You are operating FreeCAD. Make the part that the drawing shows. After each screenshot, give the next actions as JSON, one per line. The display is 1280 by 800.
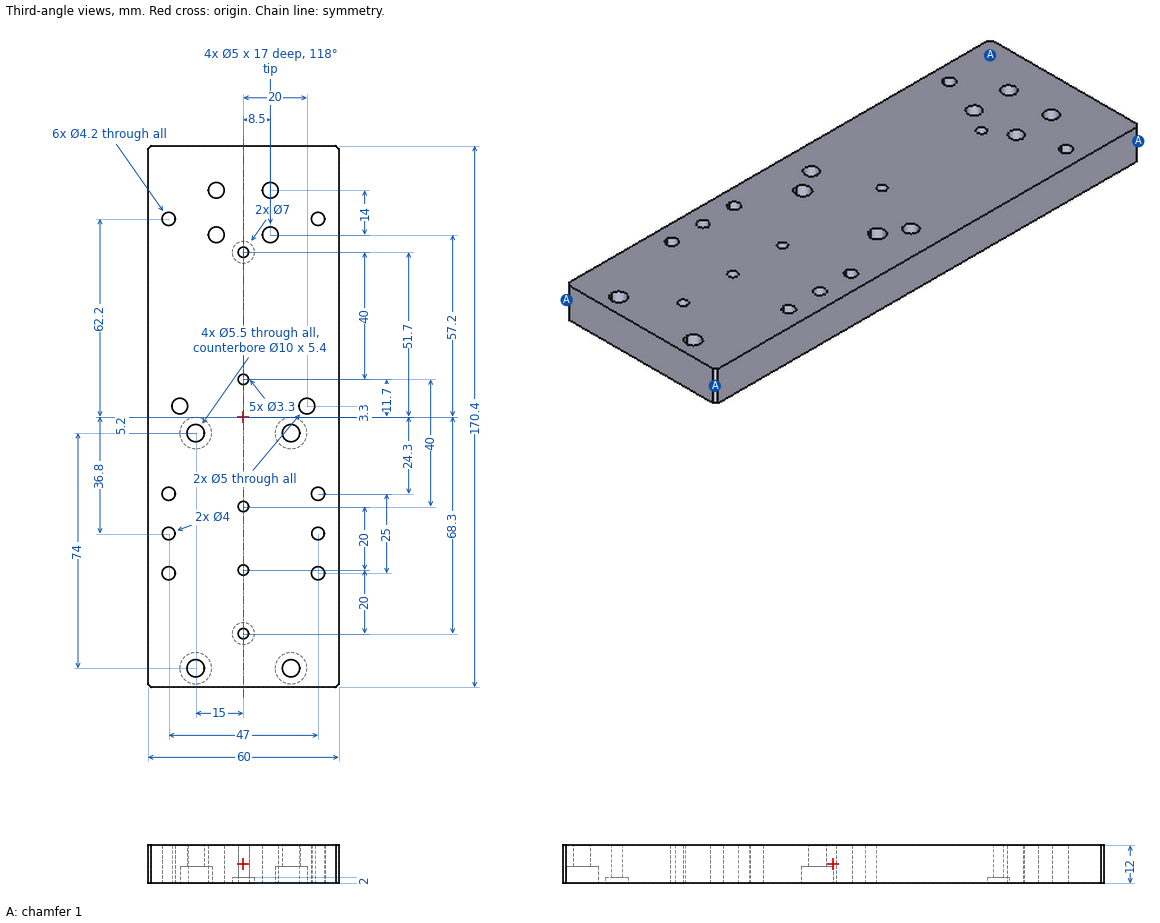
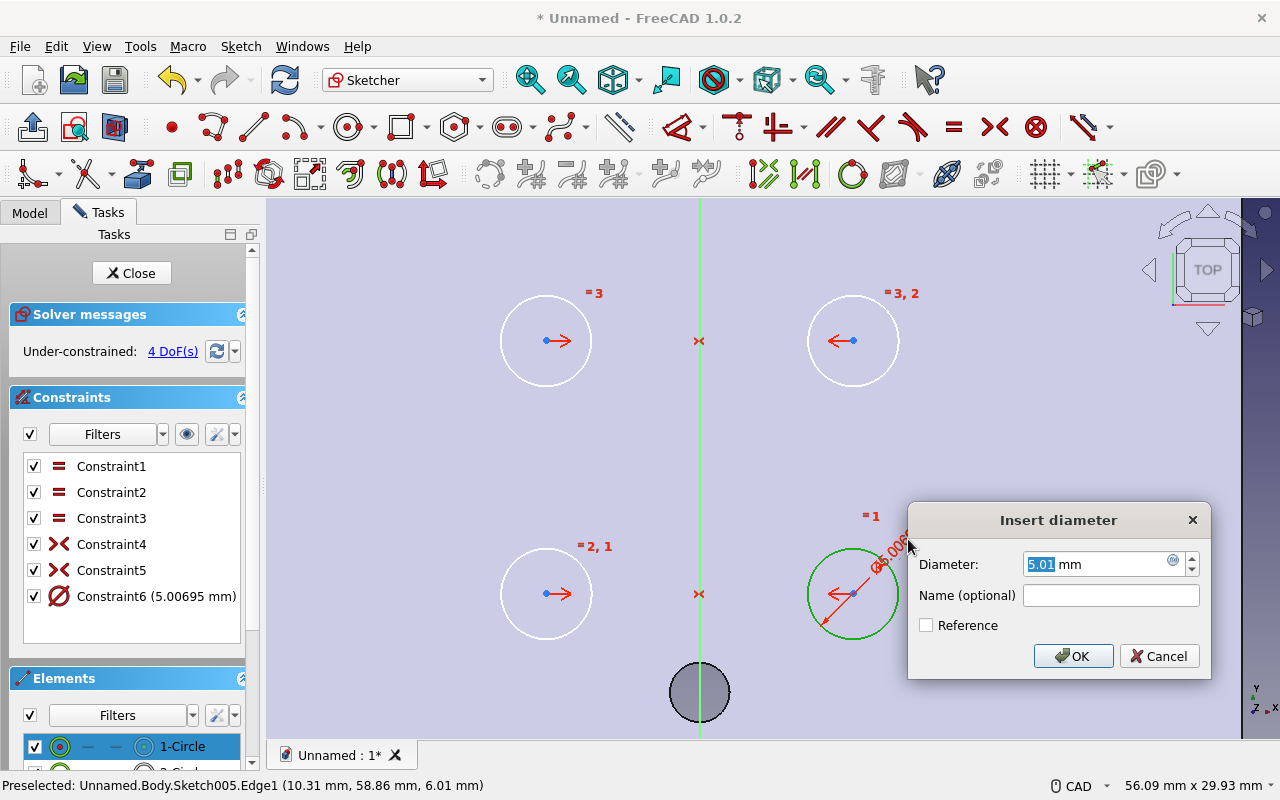
{"action": "type", "text": "5"}
{"action": "key", "text": "Return"}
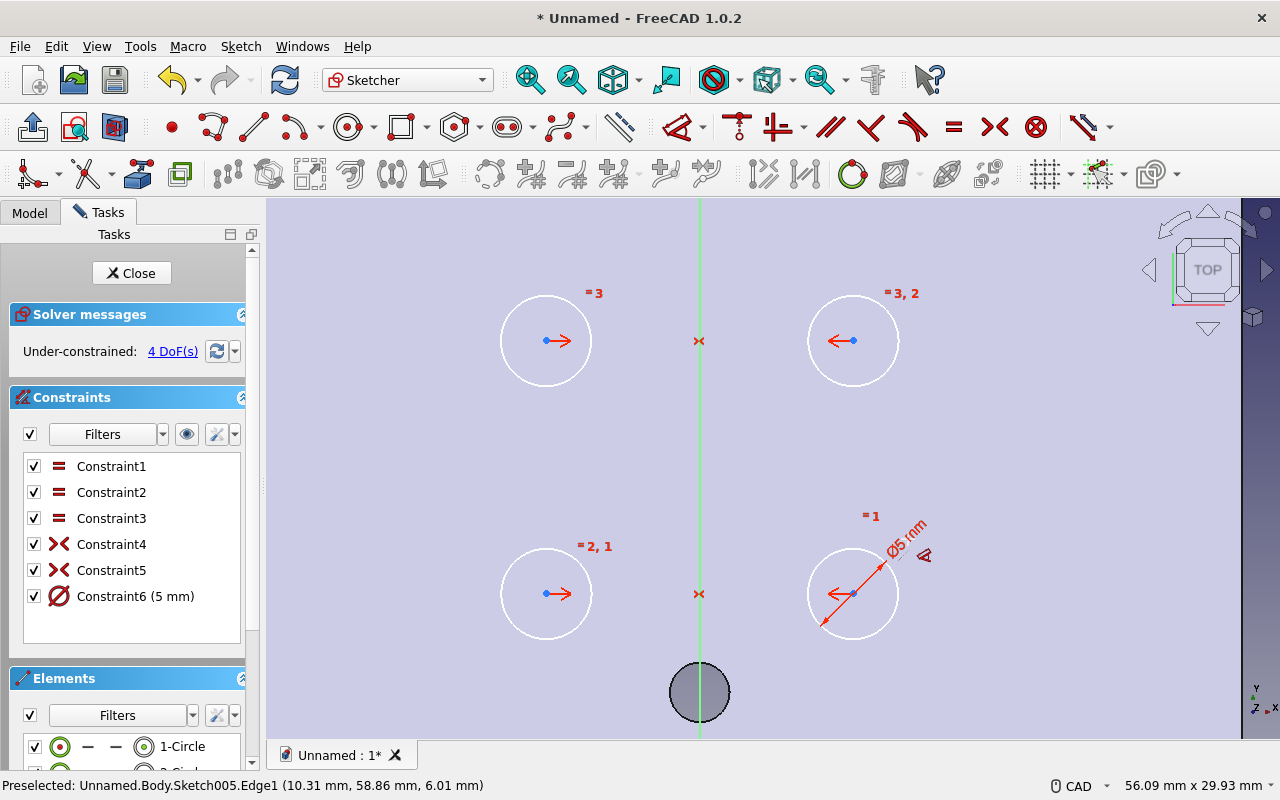
{"action": "left_click", "coordinate": [853, 594]}
{"action": "left_click", "coordinate": [776, 560]}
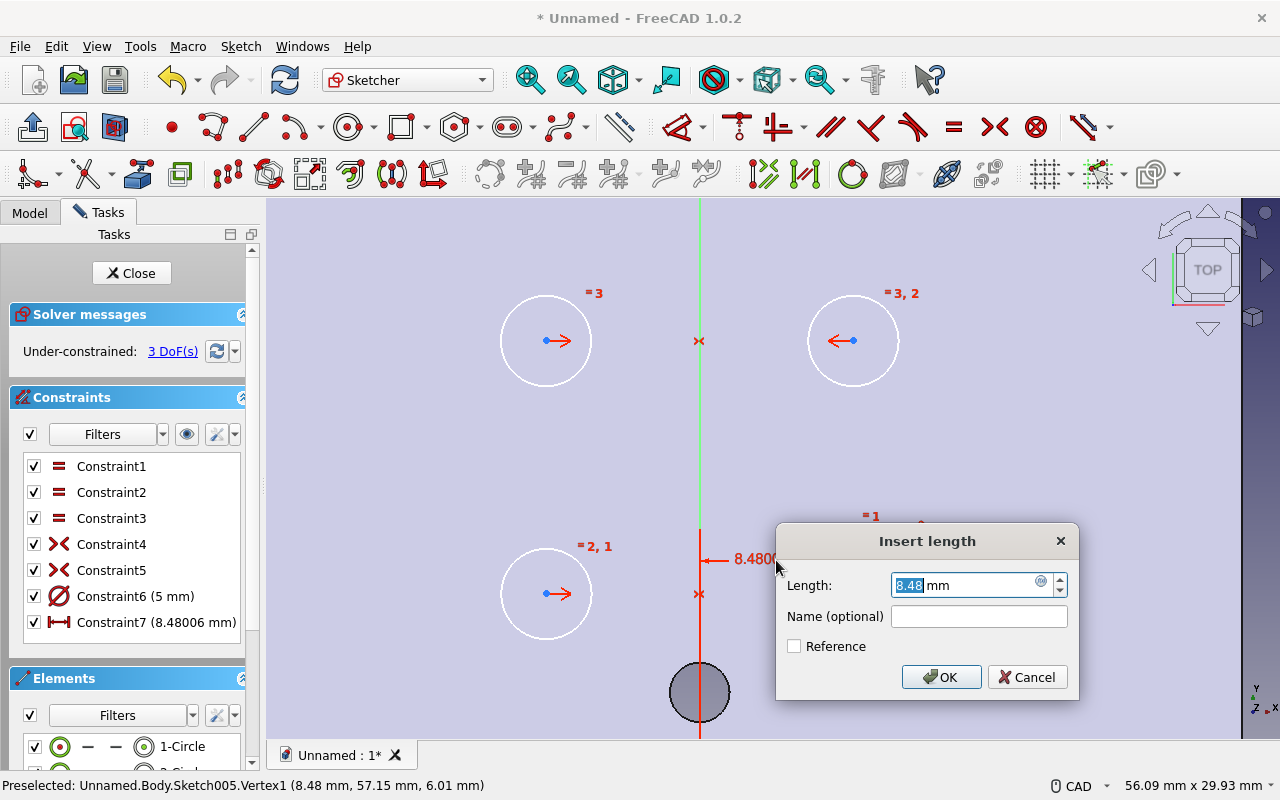
{"action": "type", "text": "8.5"}
{"action": "key", "text": "Return"}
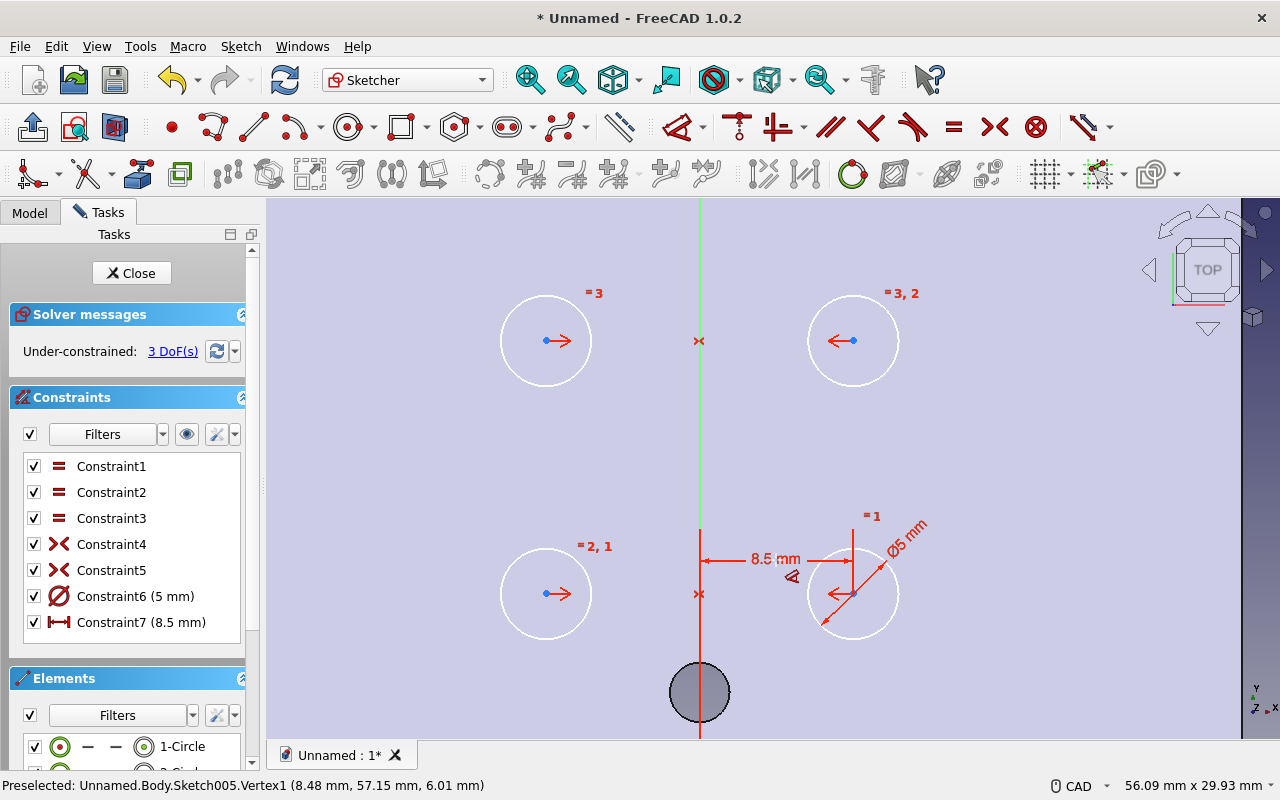
{"action": "left_click", "coordinate": [853, 341]}
{"action": "left_click", "coordinate": [777, 307]}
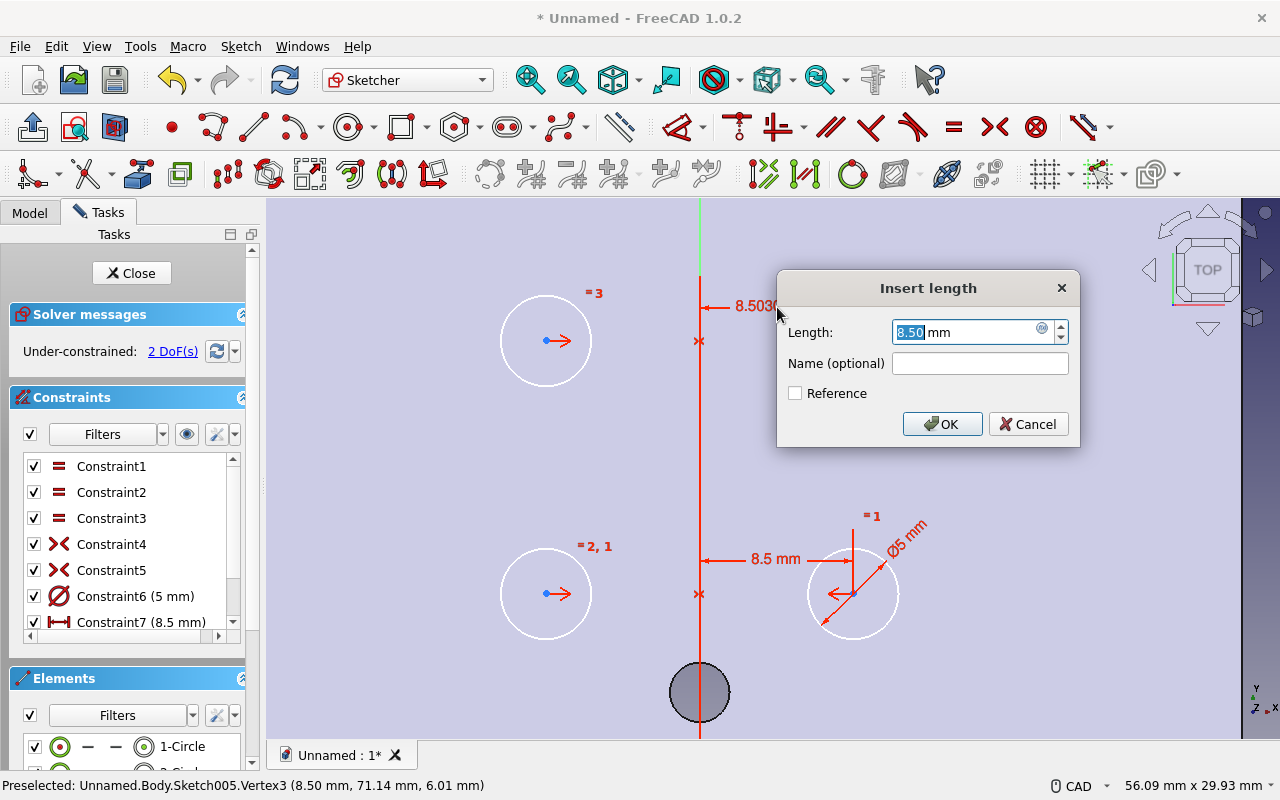
{"action": "type", "text": "8.5"}
{"action": "key", "text": "Return"}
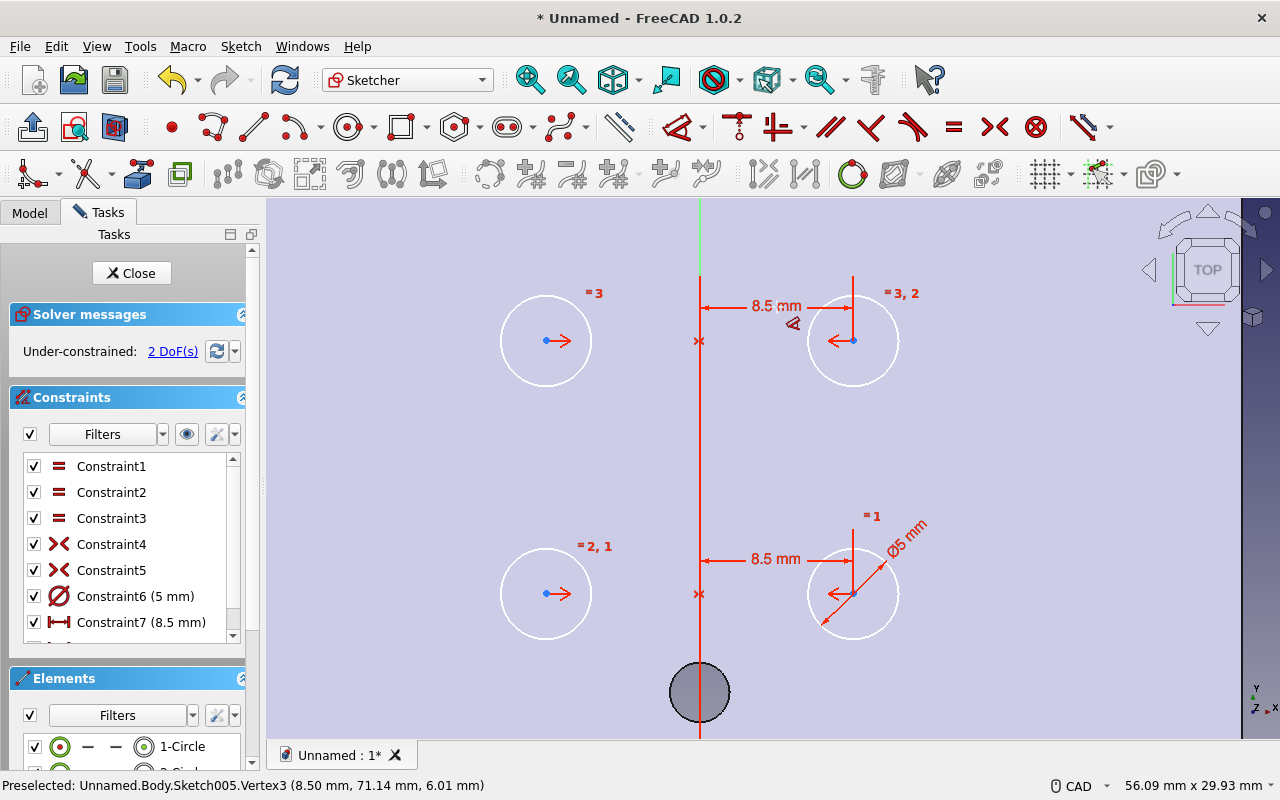
{"action": "left_click", "coordinate": [853, 594]}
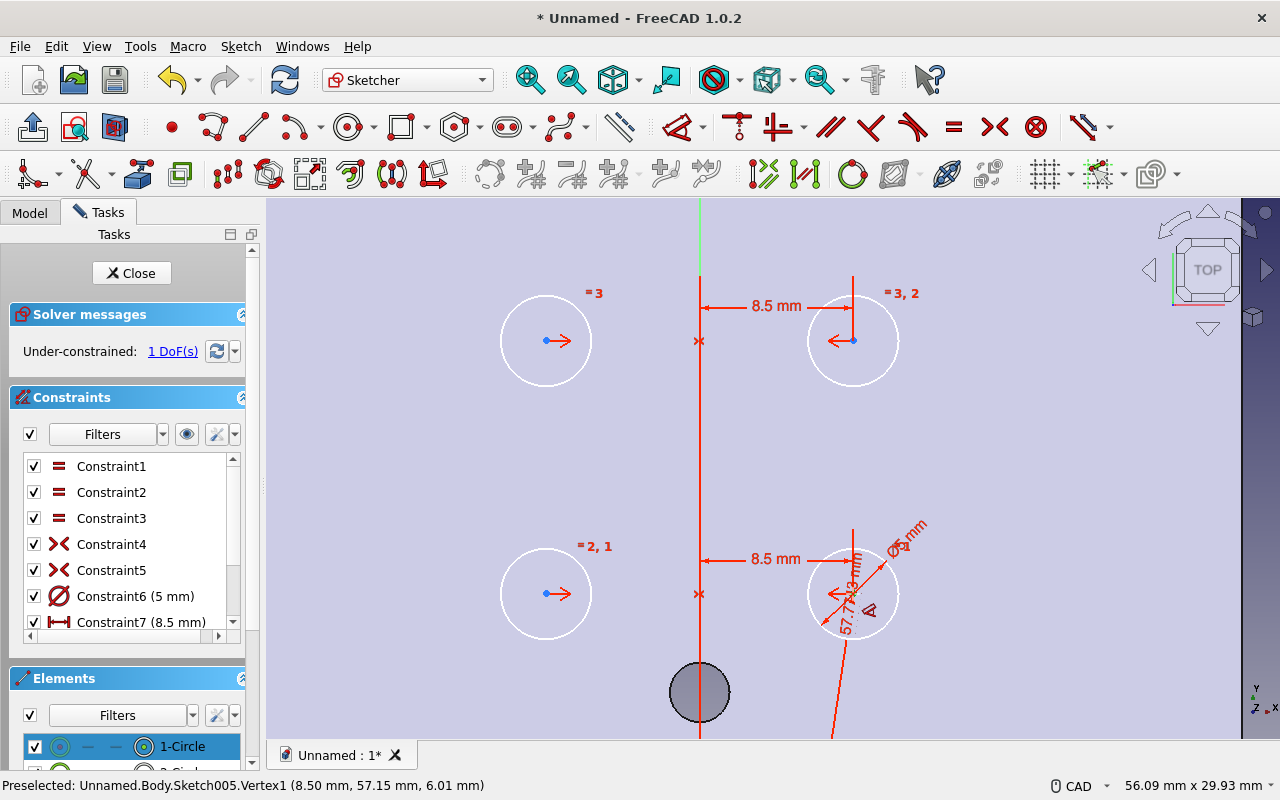
{"action": "left_click", "coordinate": [853, 341]}
{"action": "left_click", "coordinate": [887, 467]}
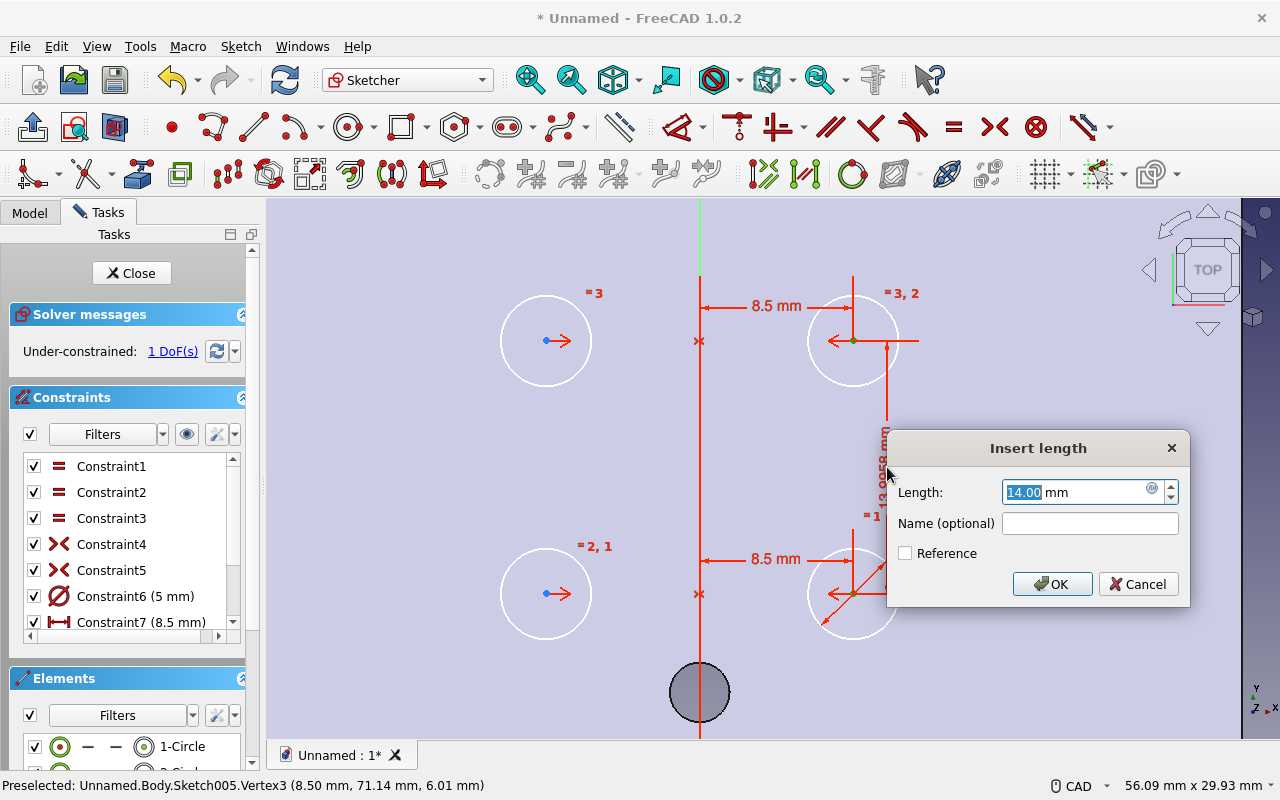
{"action": "type", "text": "14"}
{"action": "key", "text": "Return"}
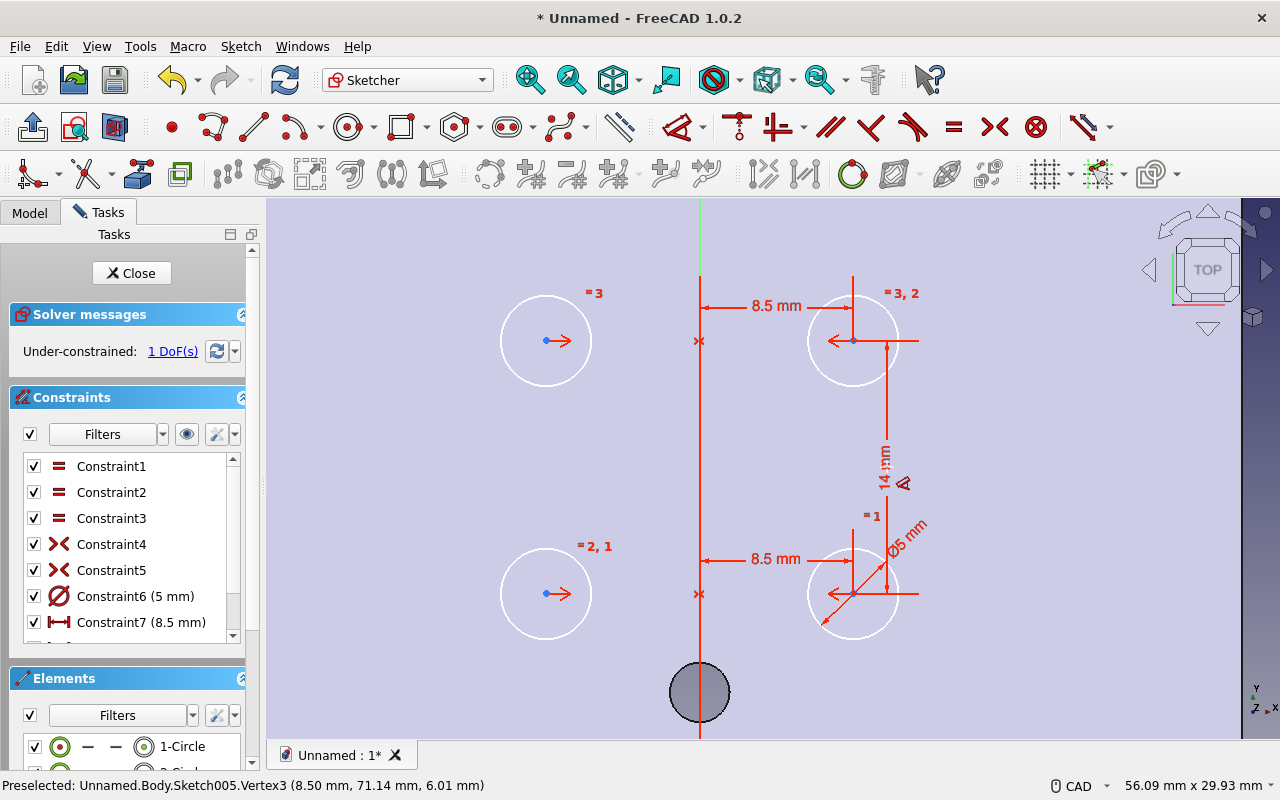
{"action": "left_click", "coordinate": [853, 594]}
{"action": "left_click", "coordinate": [887, 652]}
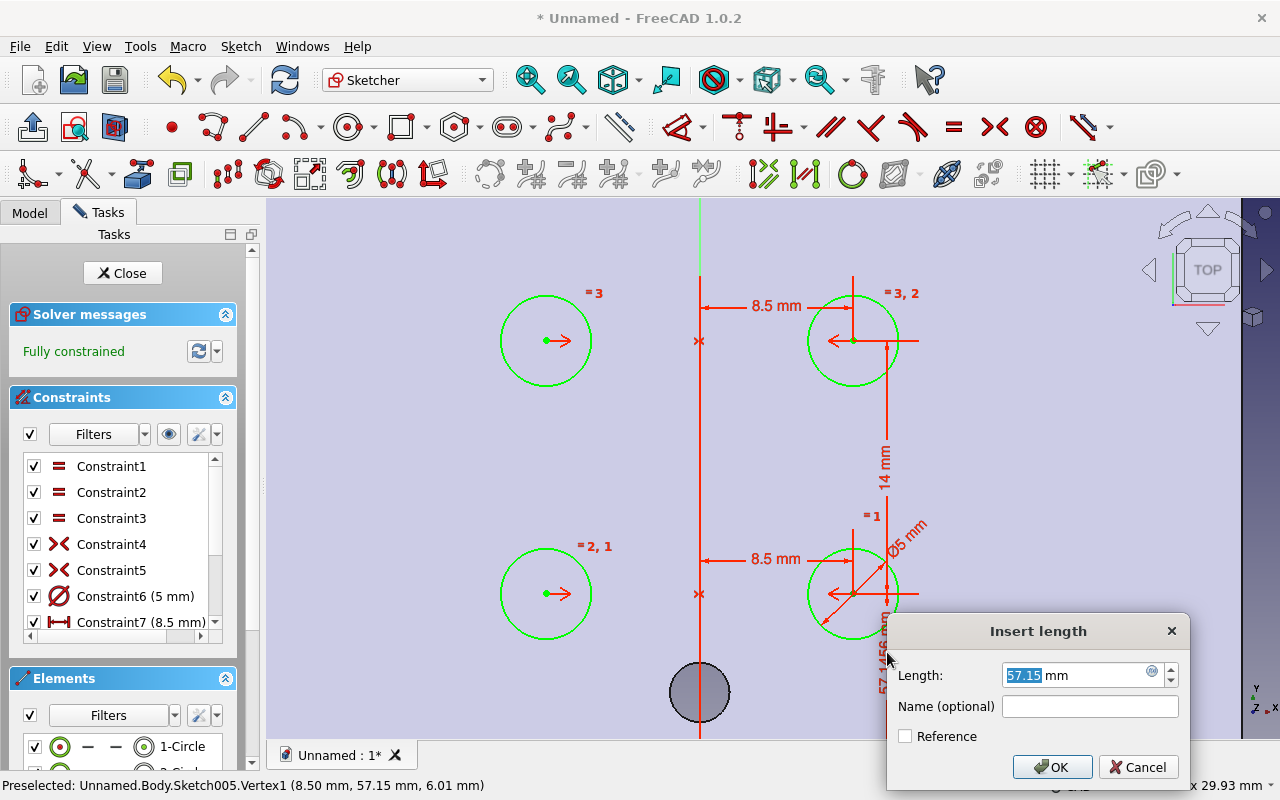
{"action": "type", "text": "57.2"}
{"action": "key", "text": "Return"}
{"action": "key", "text": "Escape"}